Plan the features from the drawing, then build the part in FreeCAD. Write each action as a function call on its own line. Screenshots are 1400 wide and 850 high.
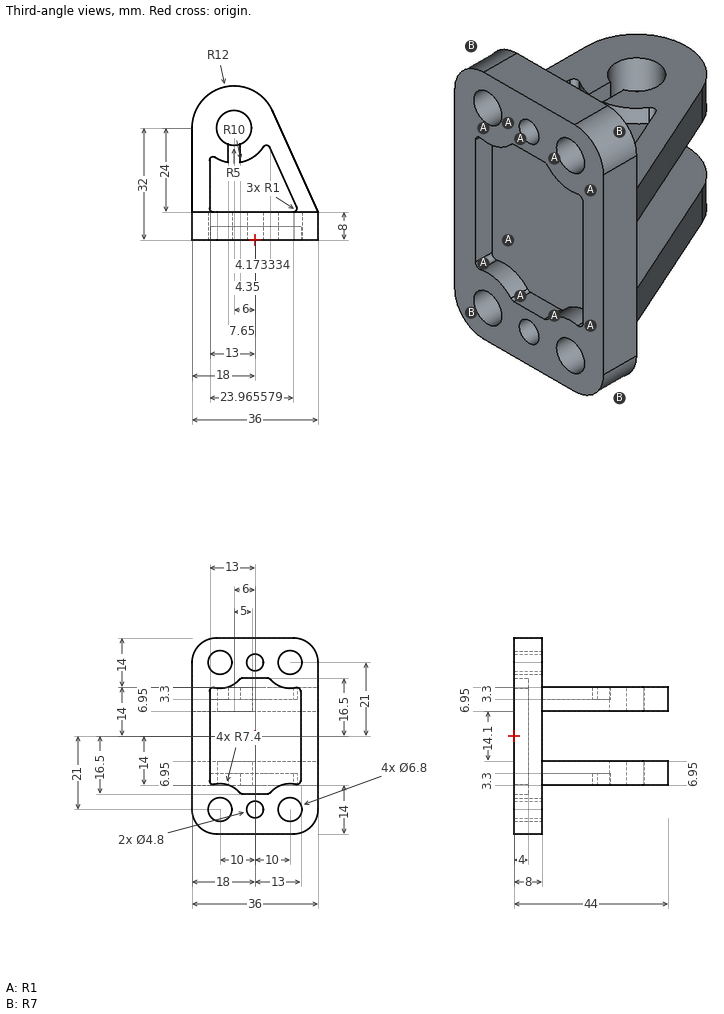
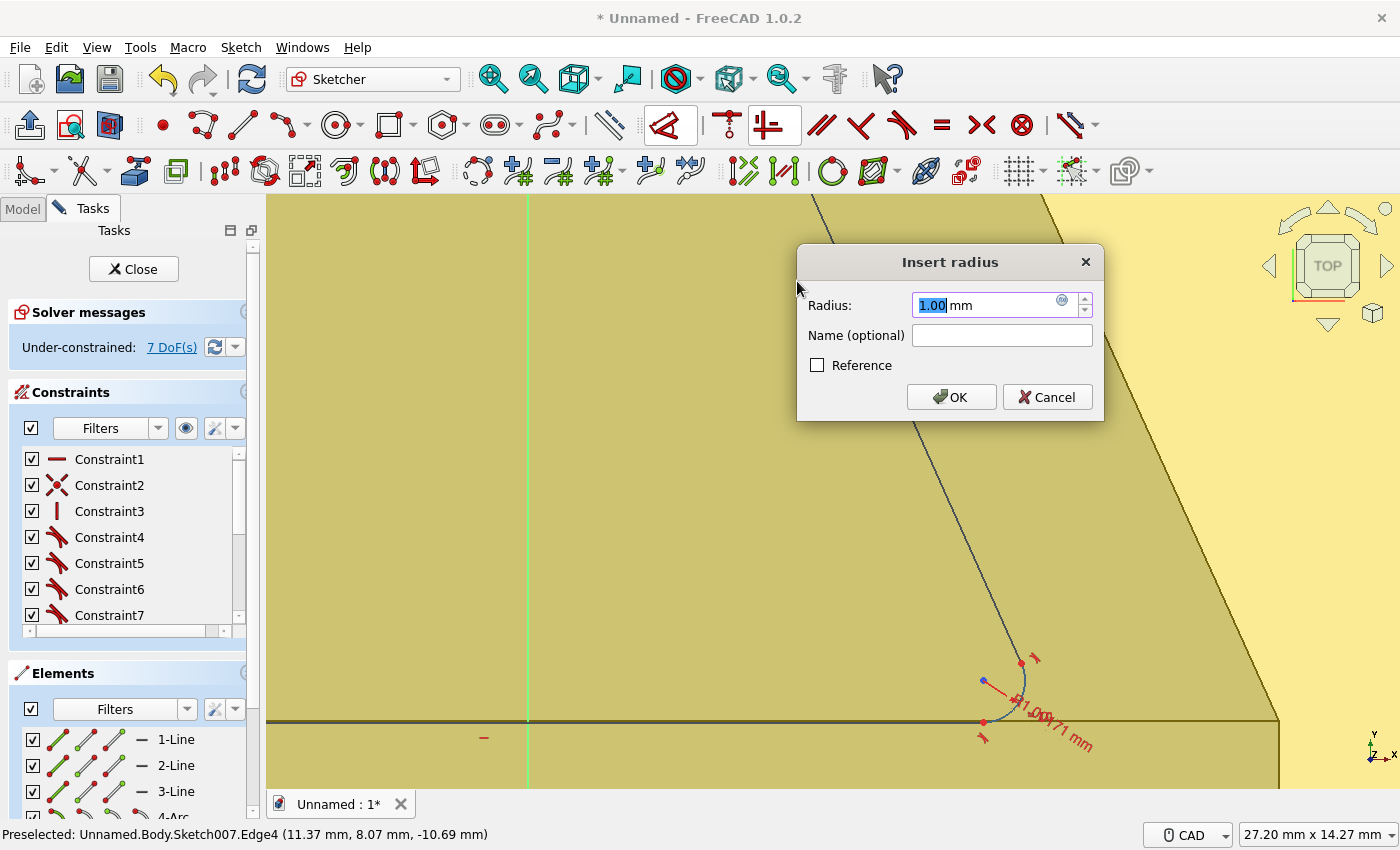
text(1)
key(Return)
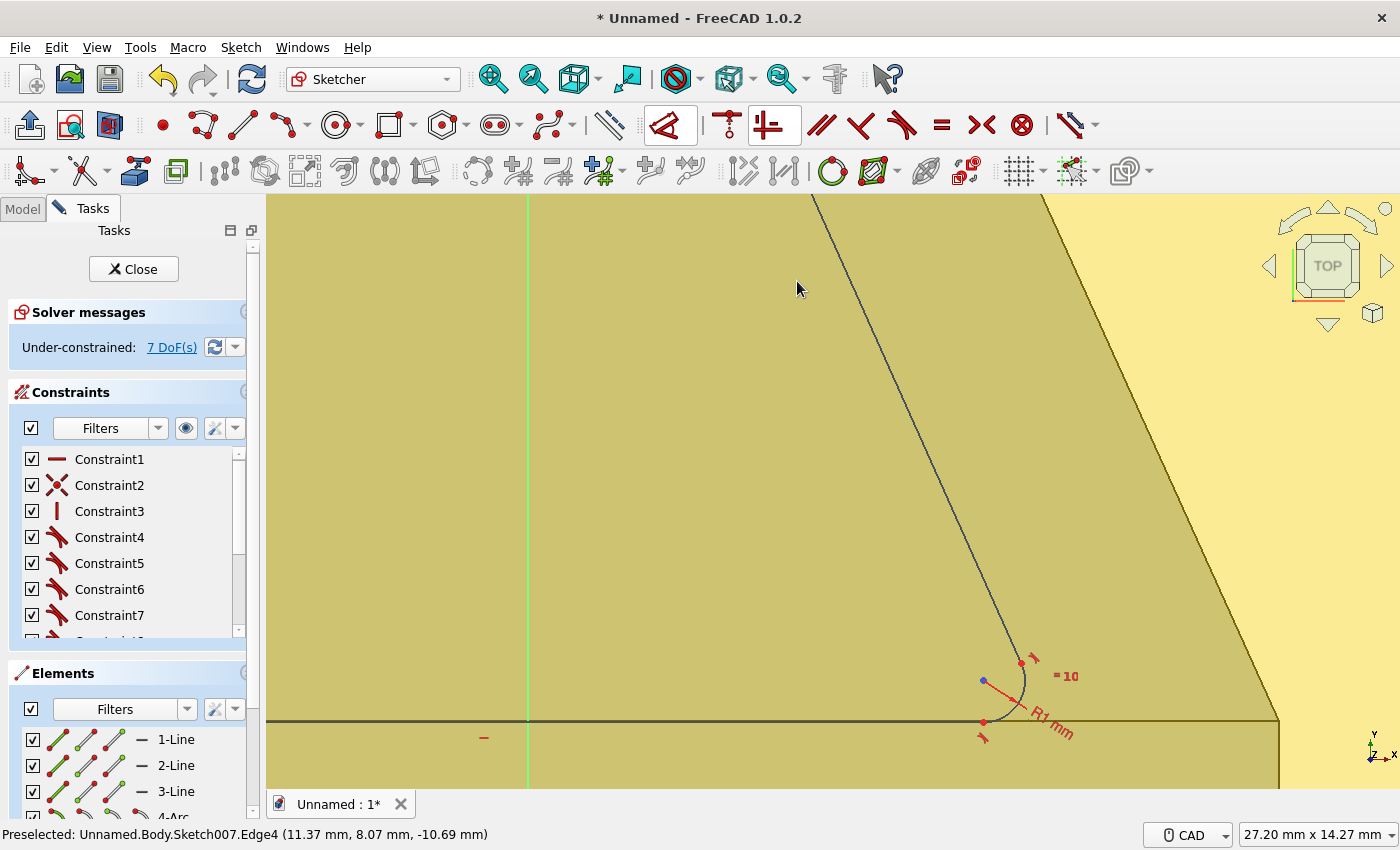
scroll(916, 492, down, 5)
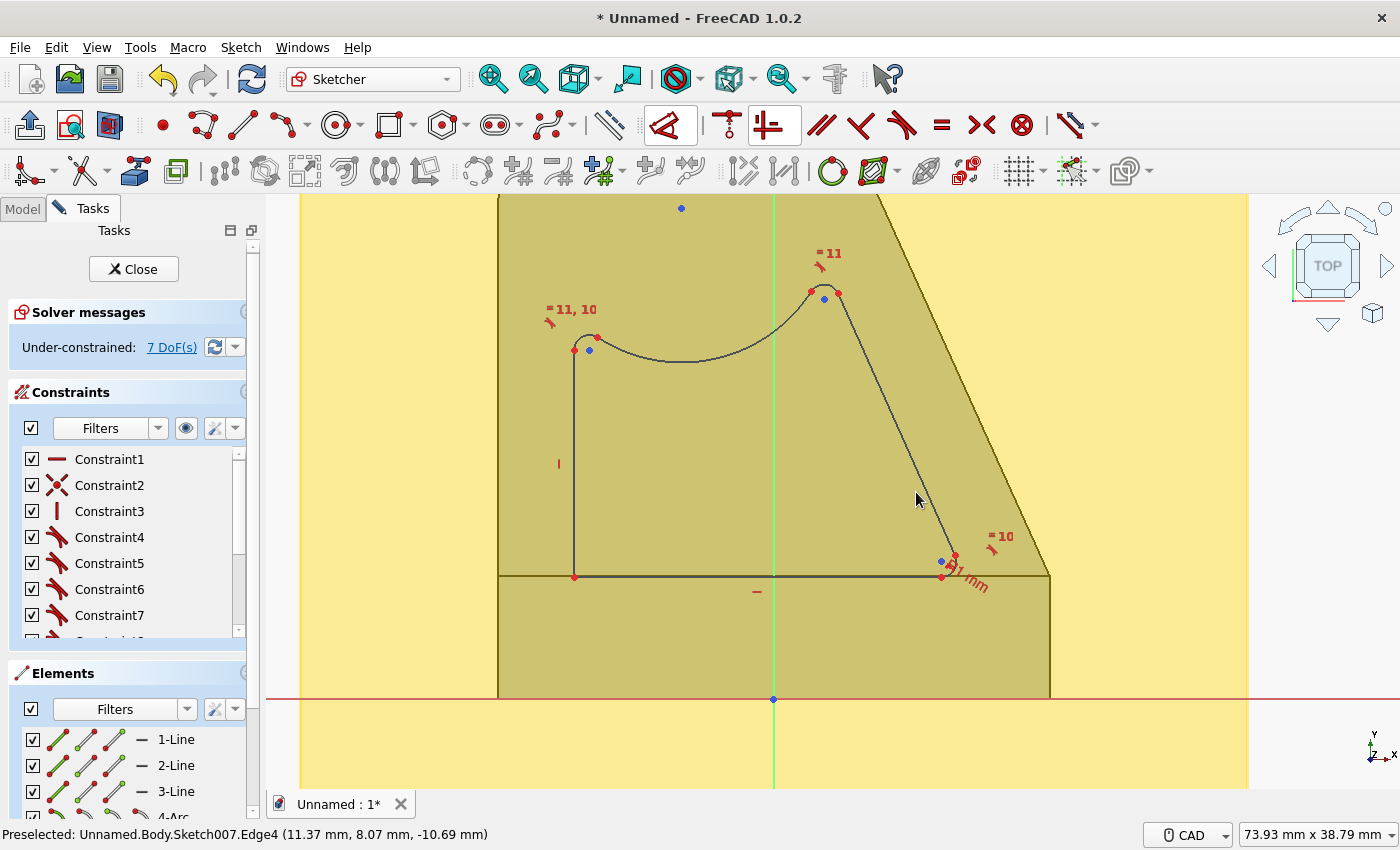
click(666, 362)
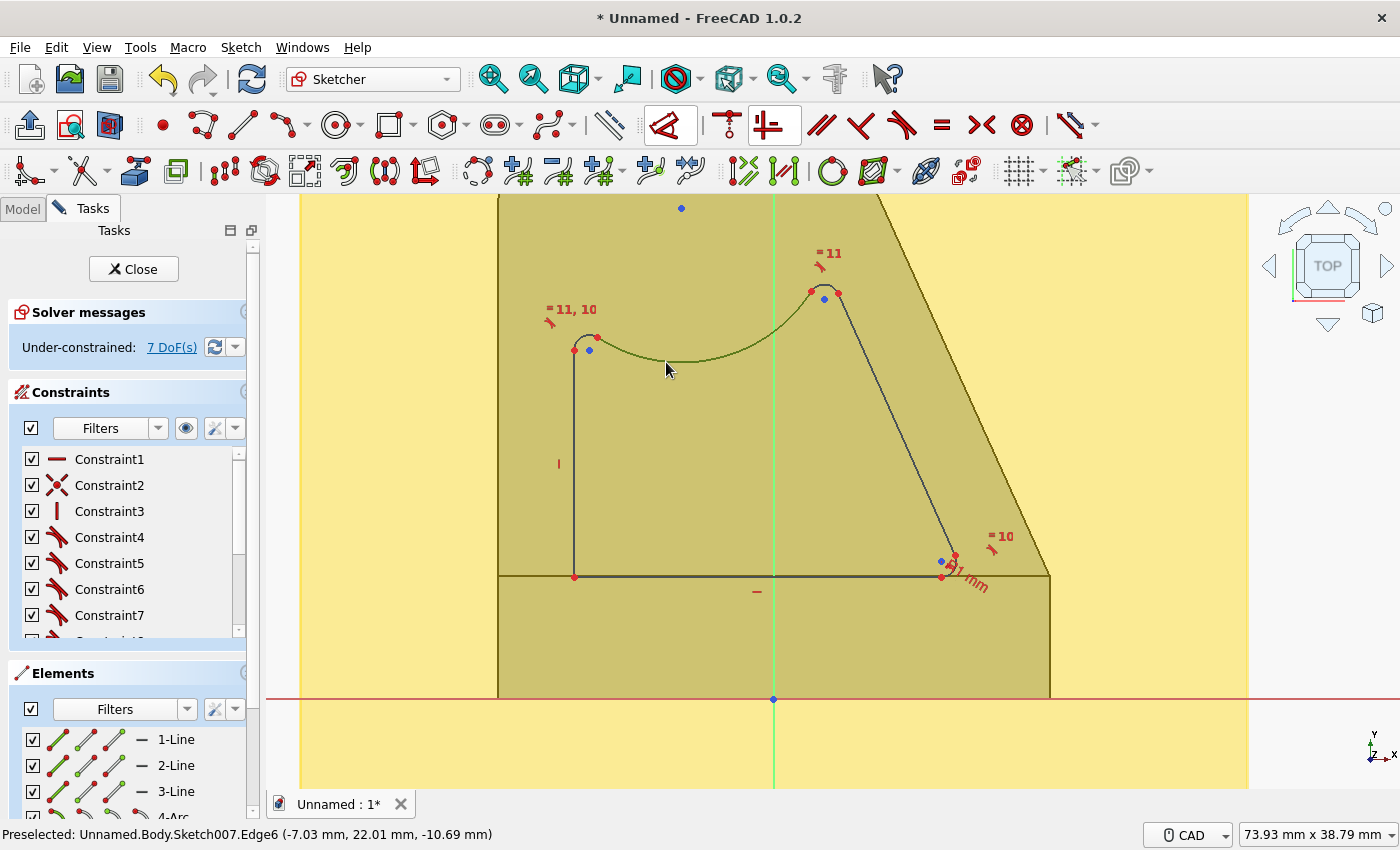
click(692, 126)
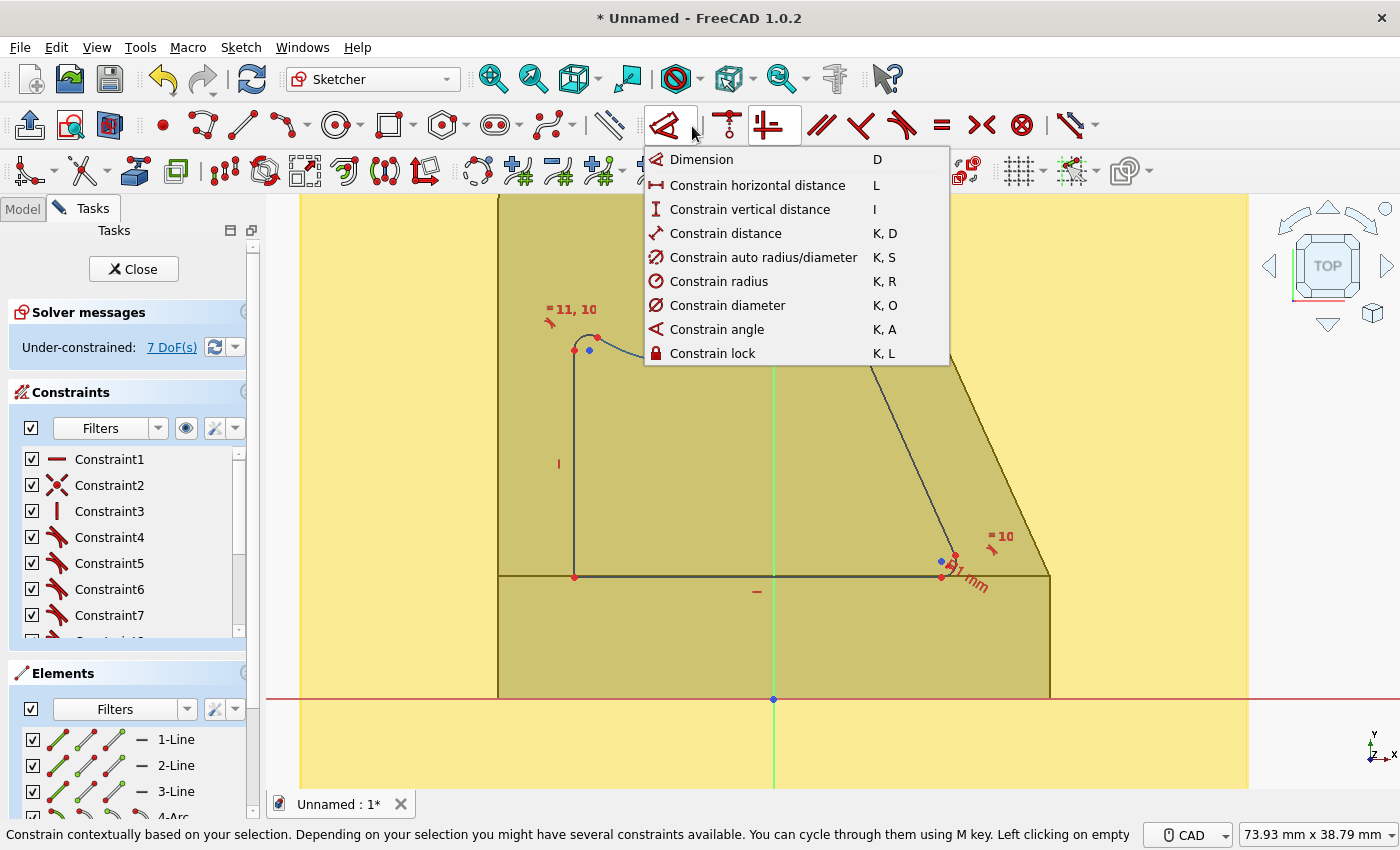
click(797, 281)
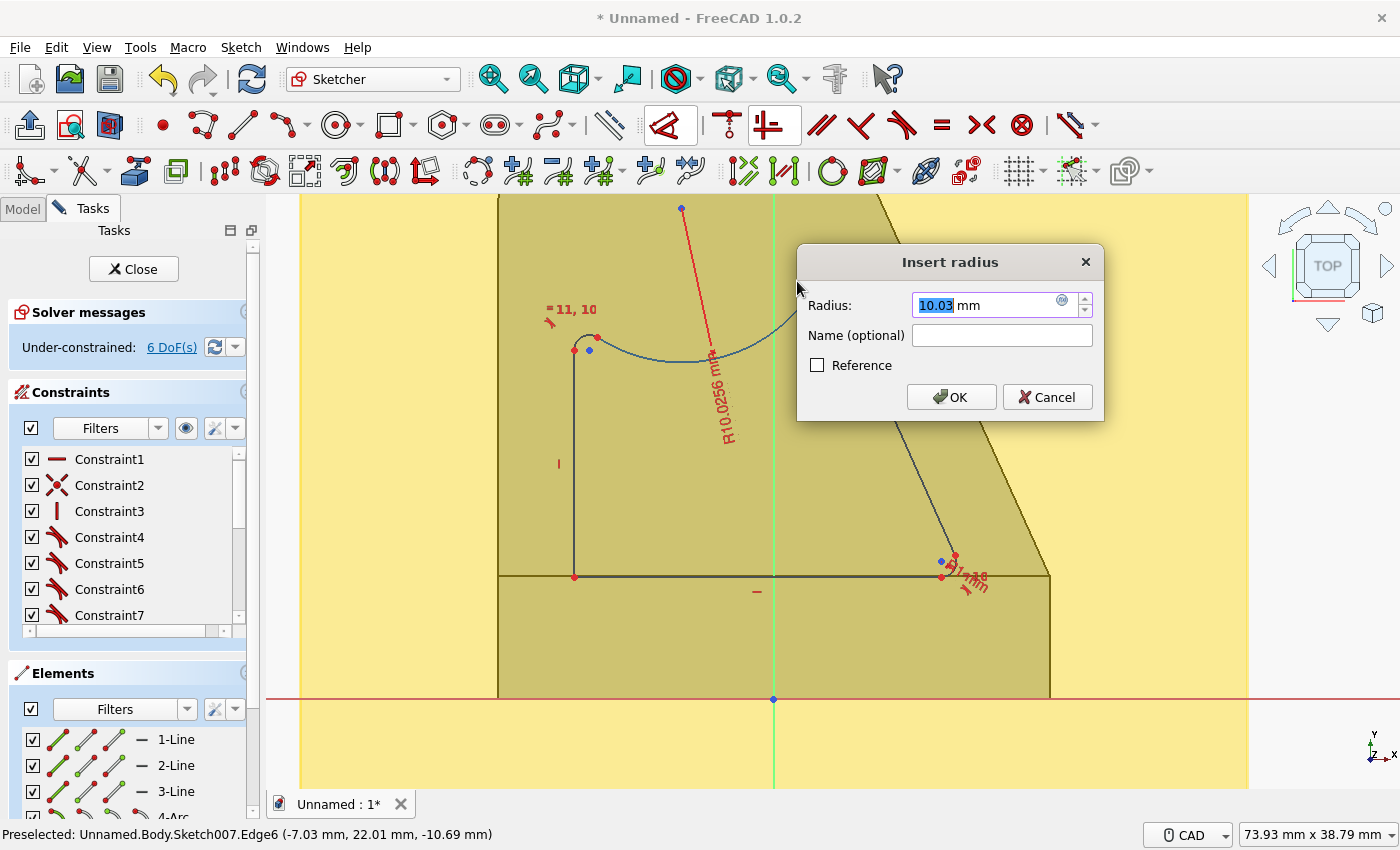
text(10)
key(Return)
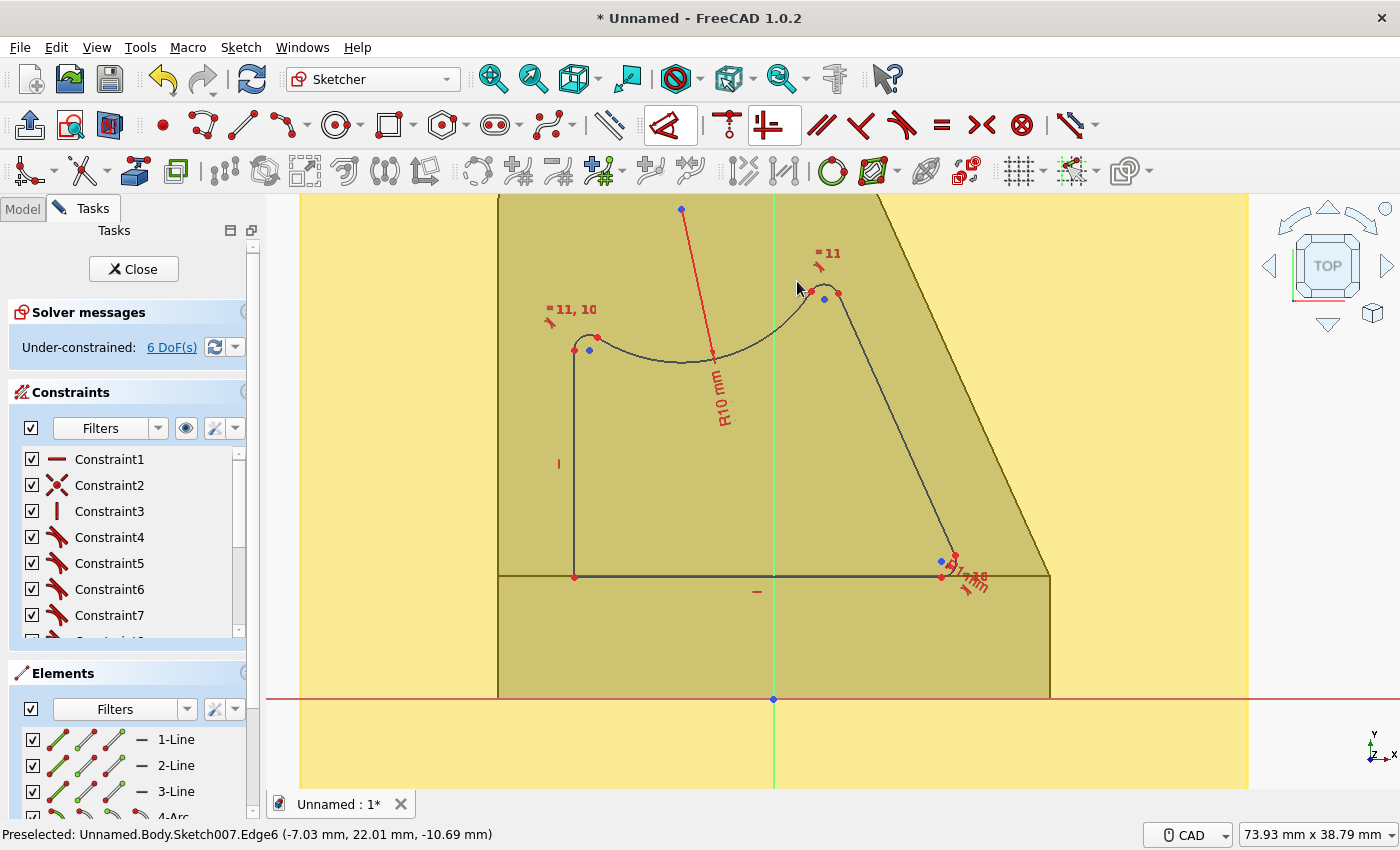
click(941, 577)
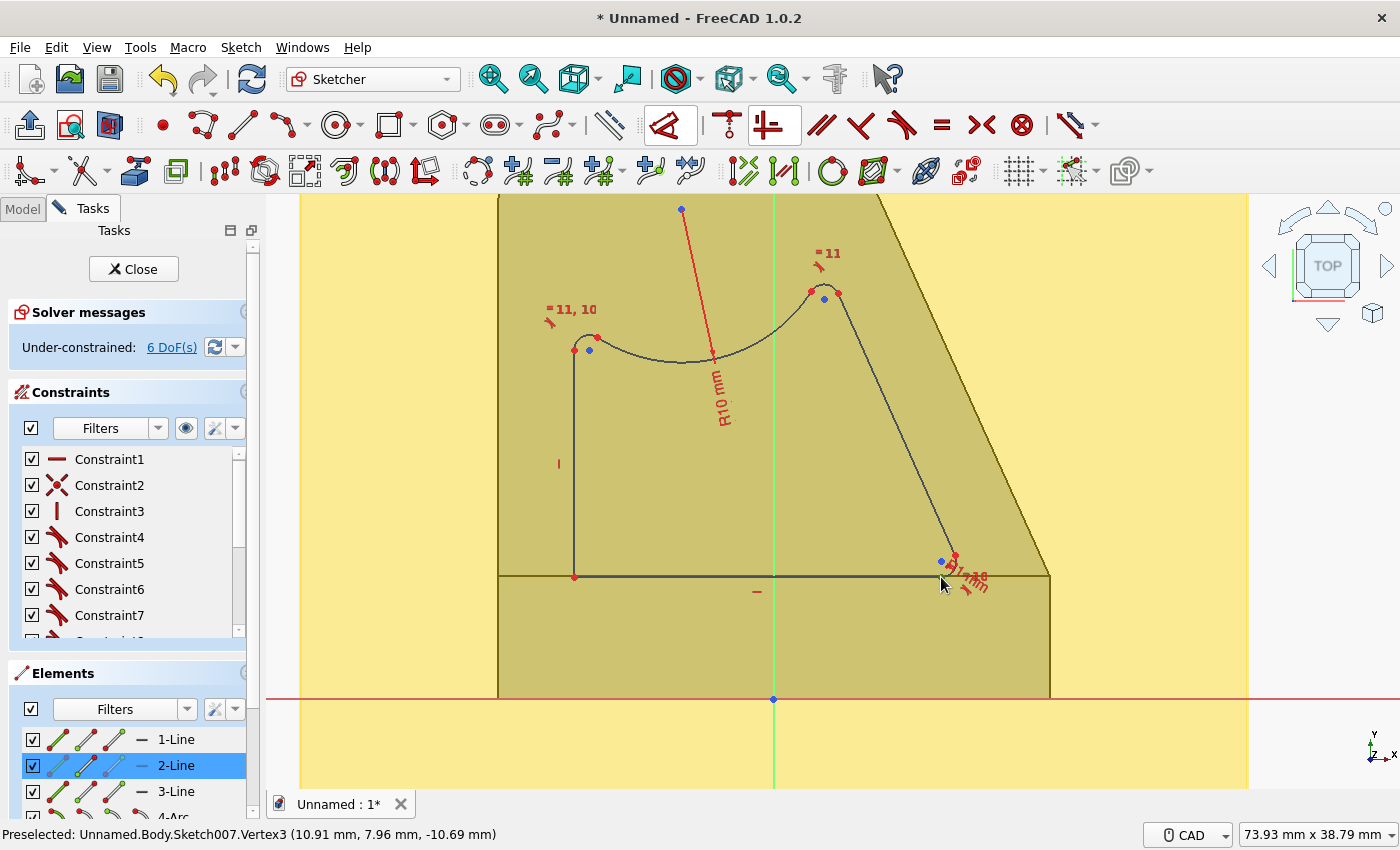
key(i)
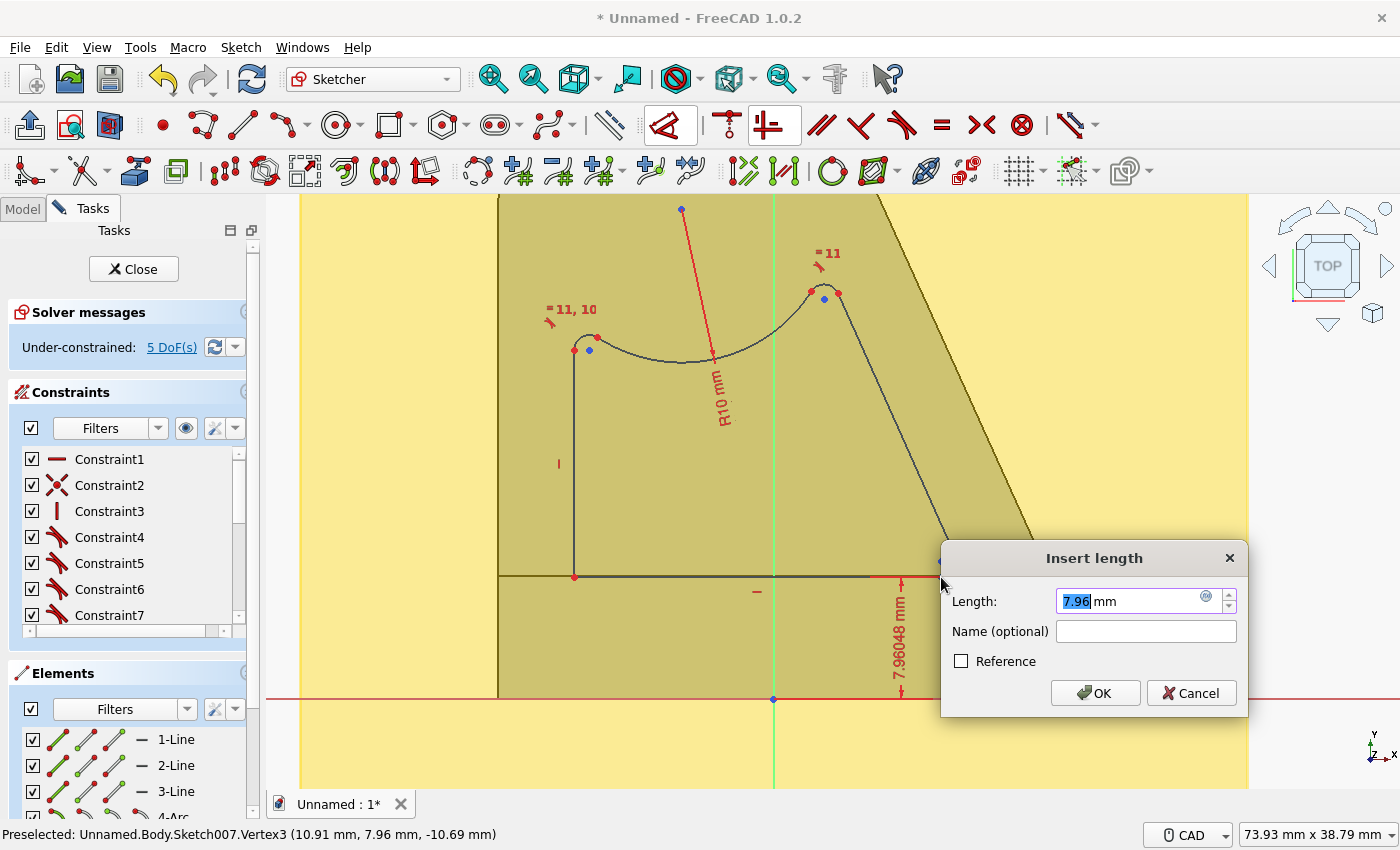
text(8)
key(Return)